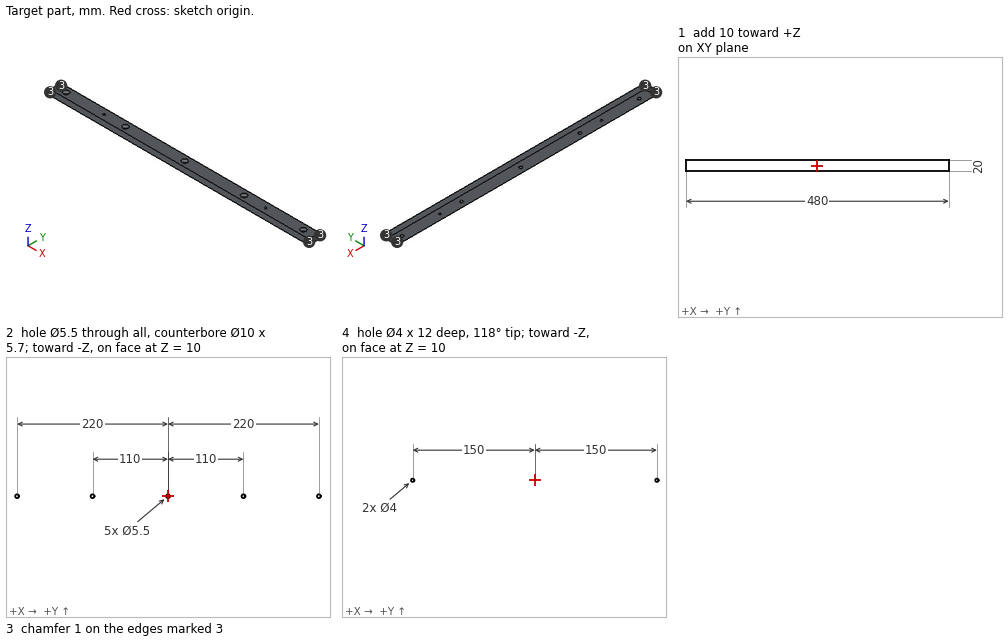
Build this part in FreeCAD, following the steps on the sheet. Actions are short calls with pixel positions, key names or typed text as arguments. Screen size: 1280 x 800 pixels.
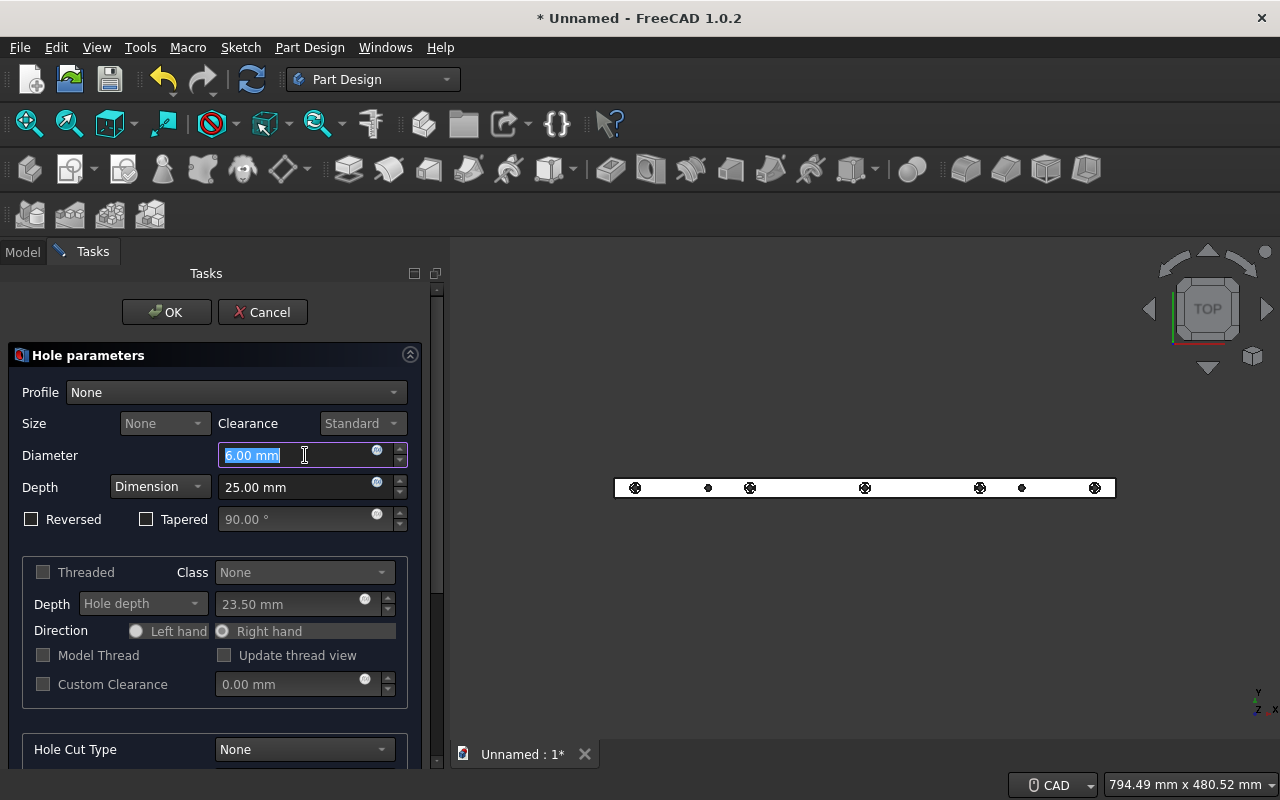
text(4)
key(Tab)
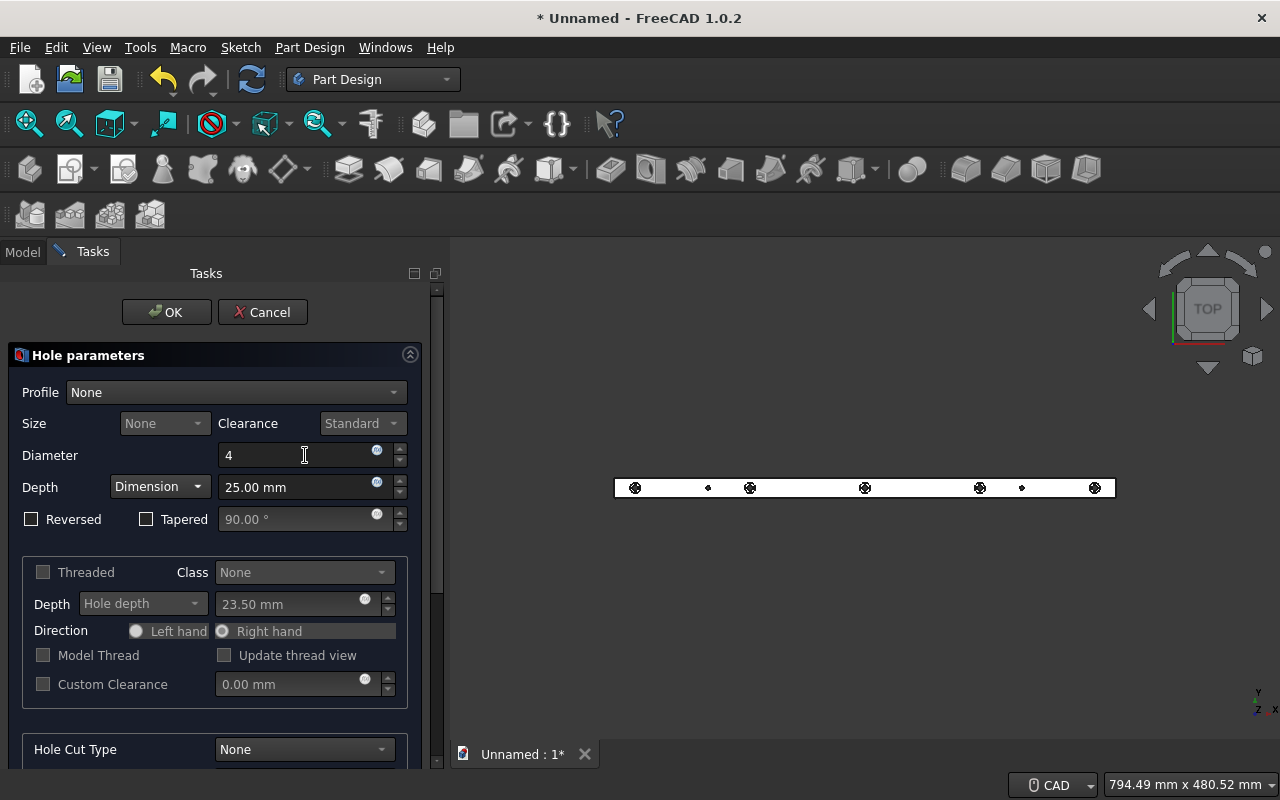
triple_click(305, 487)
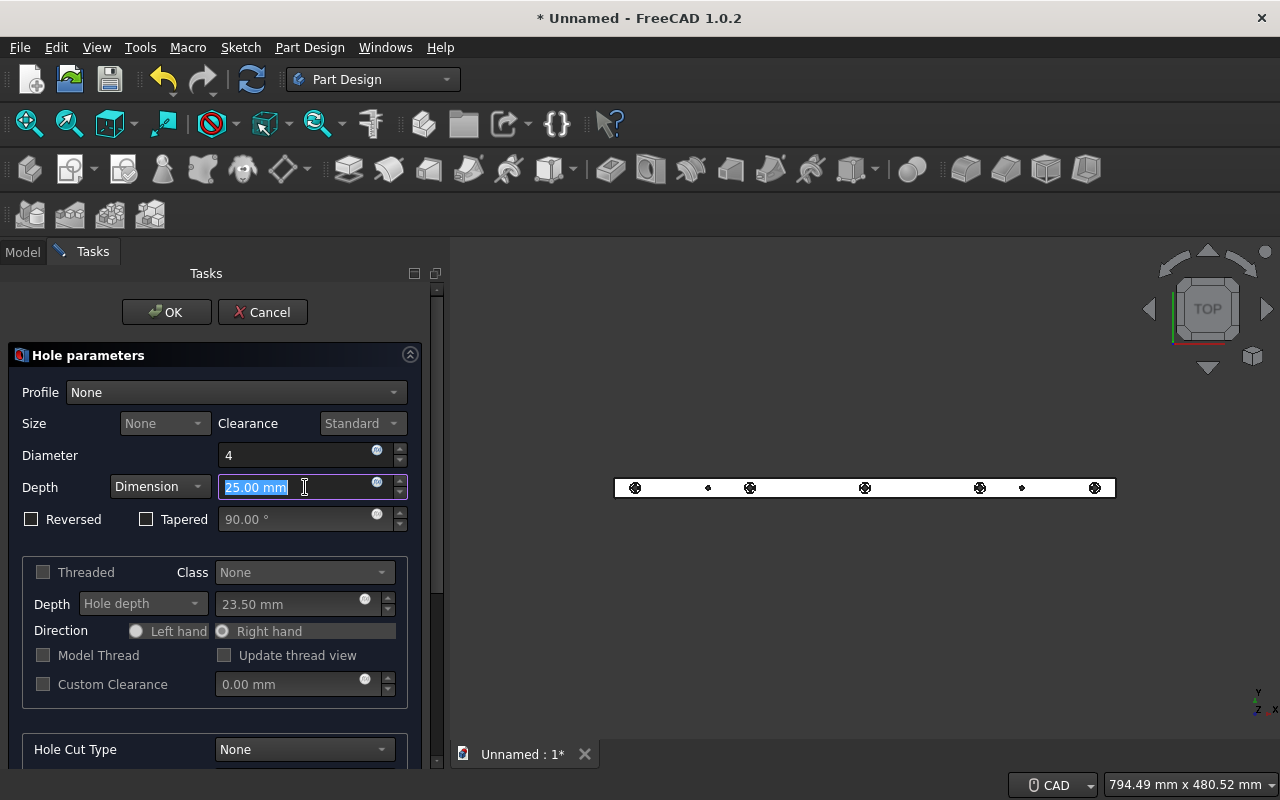
text(12)
key(Tab)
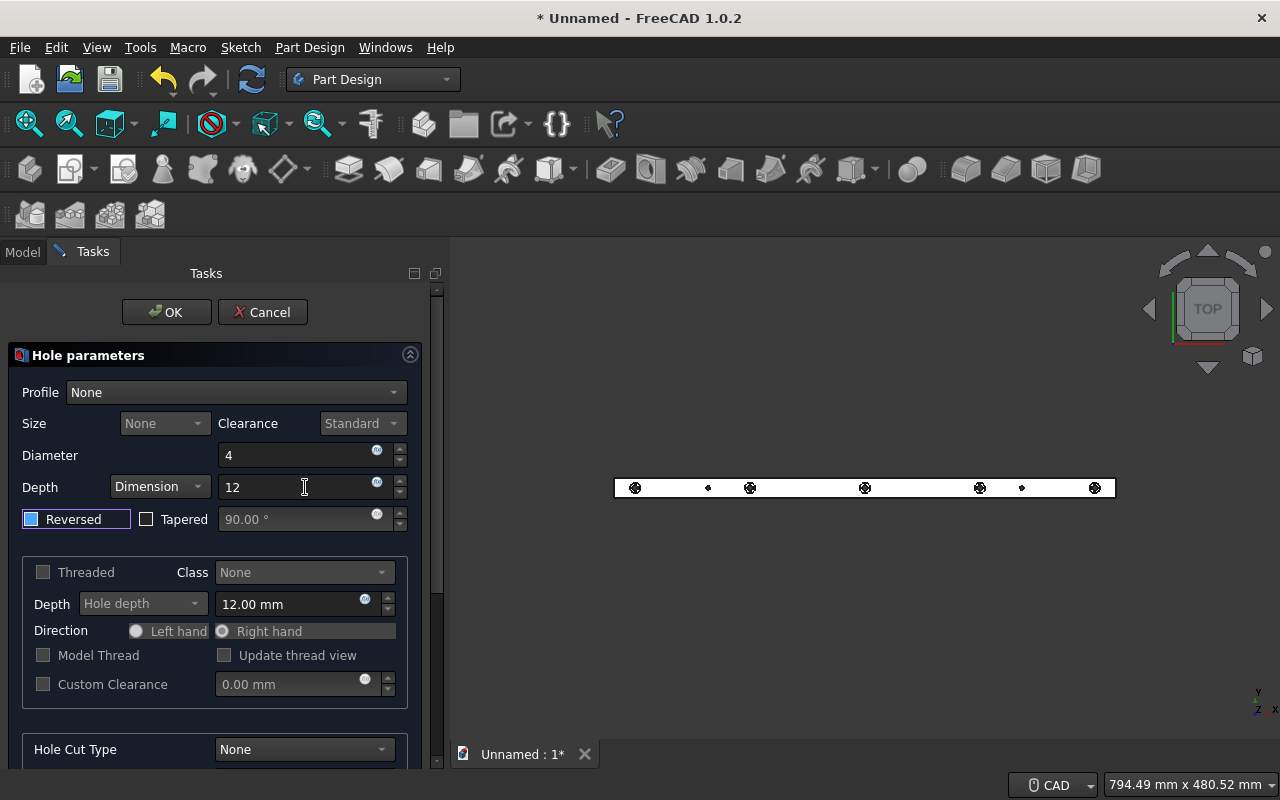
click(167, 312)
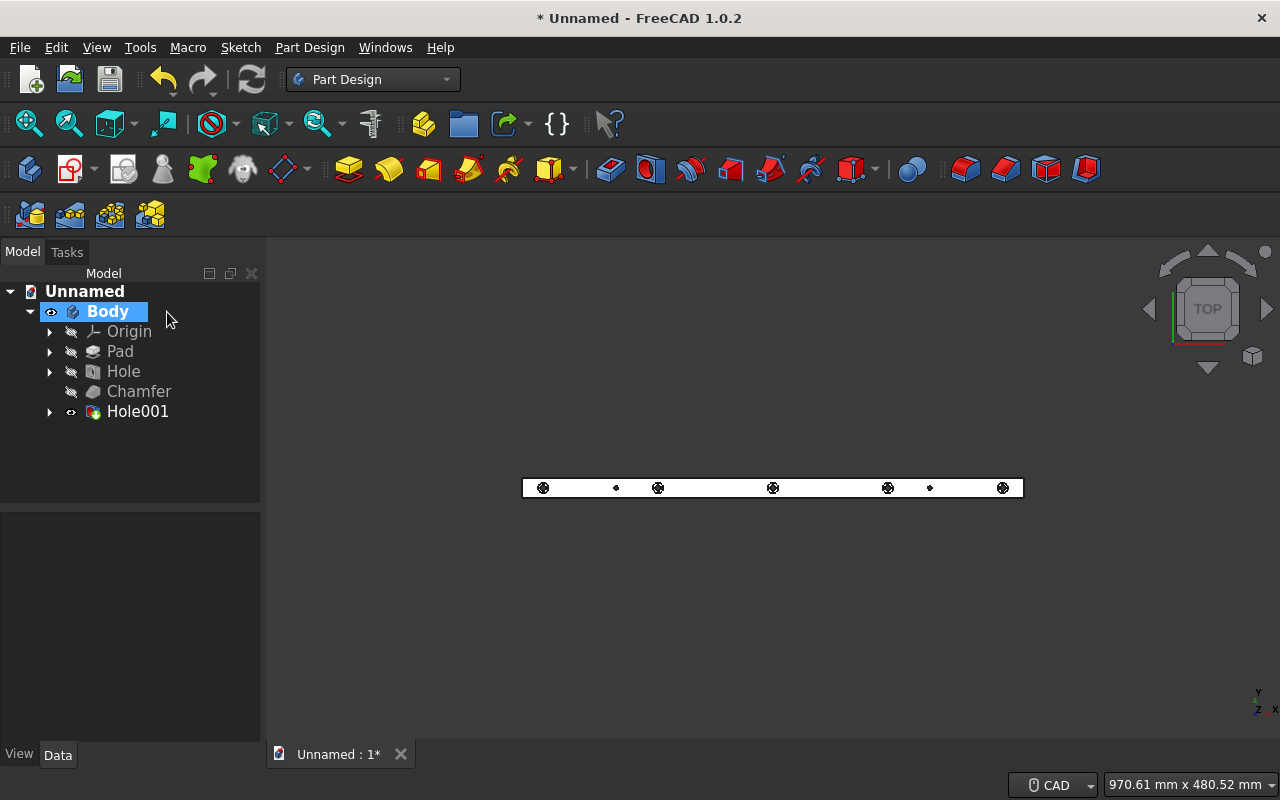
key(0)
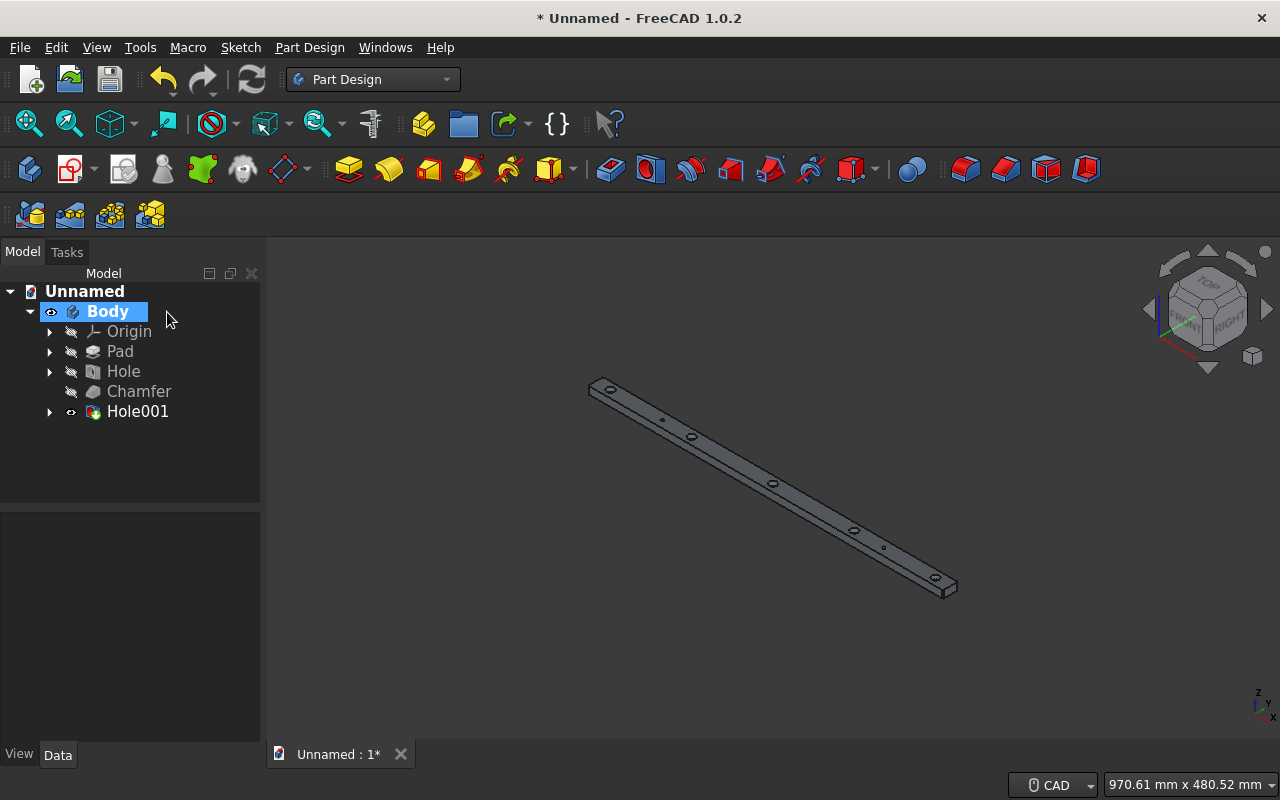
click(30, 124)